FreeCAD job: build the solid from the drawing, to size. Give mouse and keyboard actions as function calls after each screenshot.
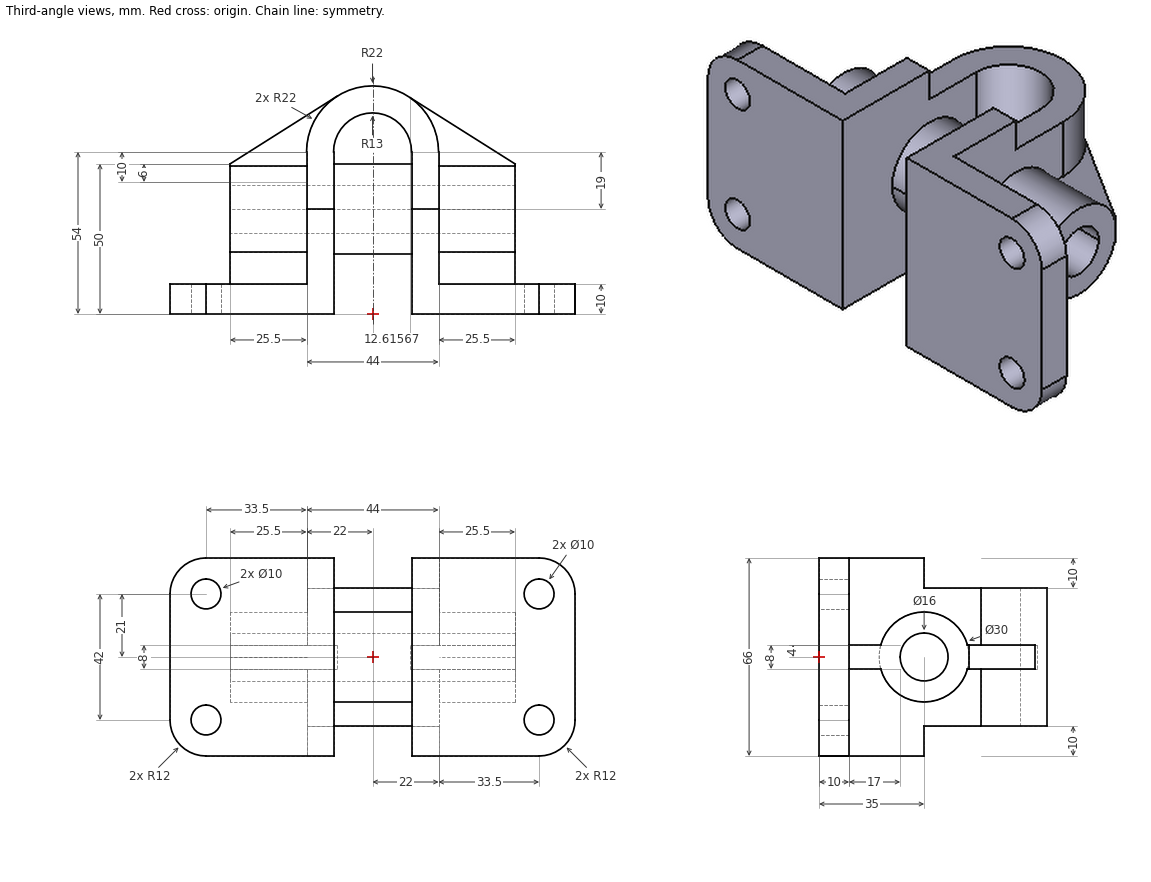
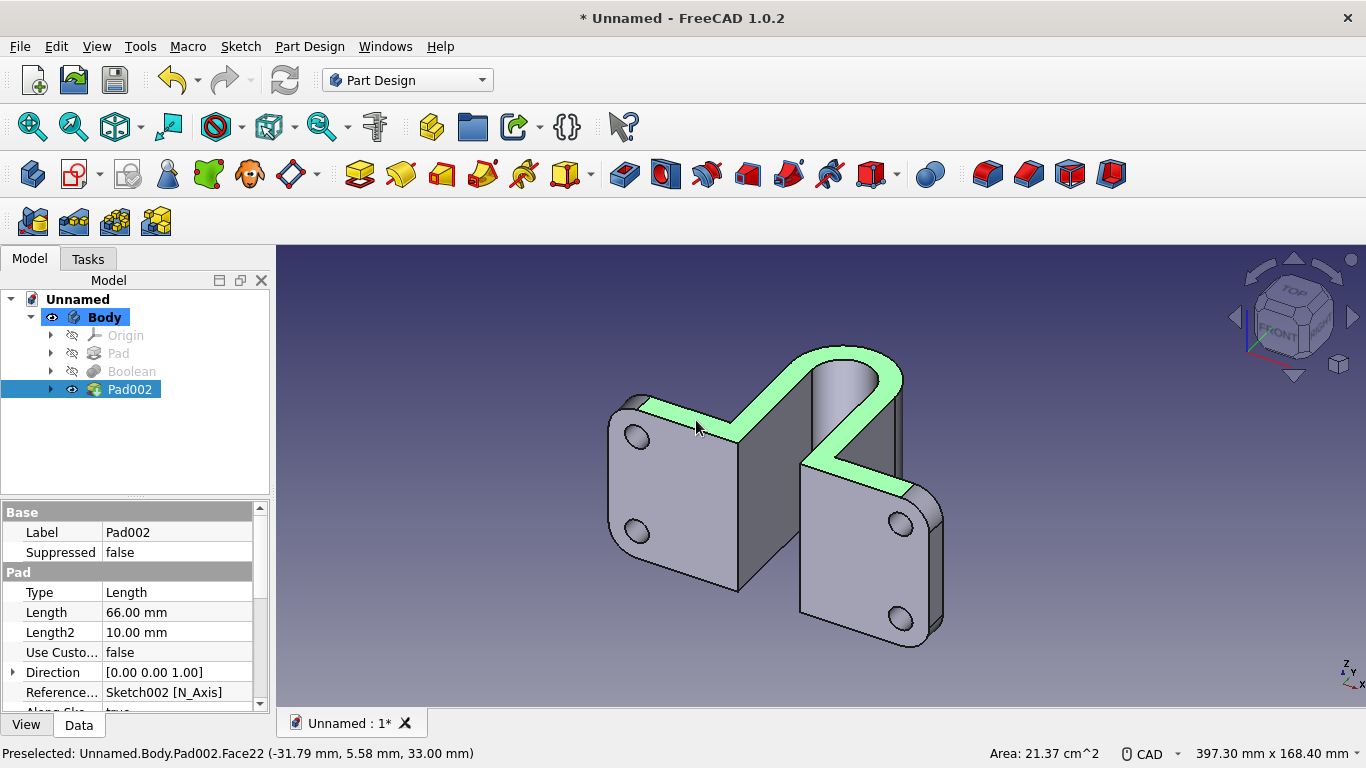
click(74, 174)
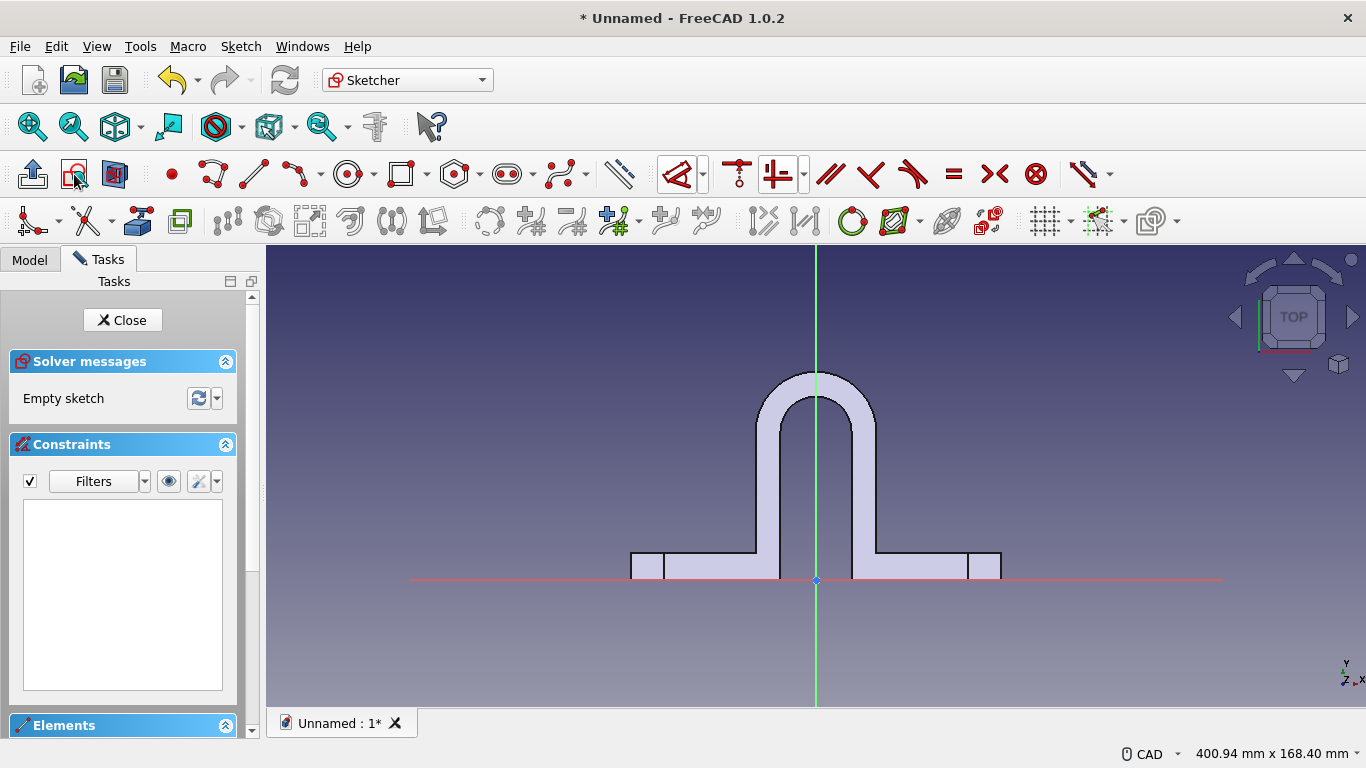
scroll(955, 476, up, 2)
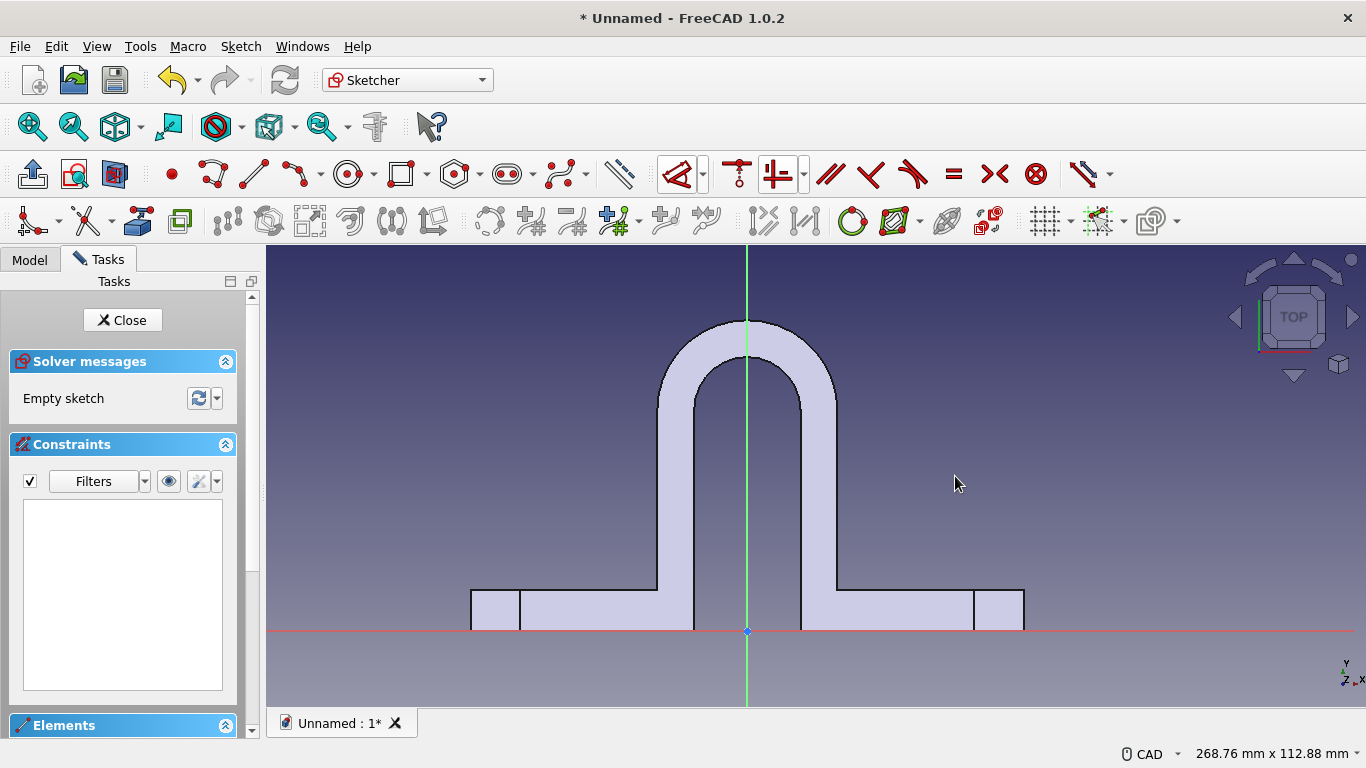
click(213, 174)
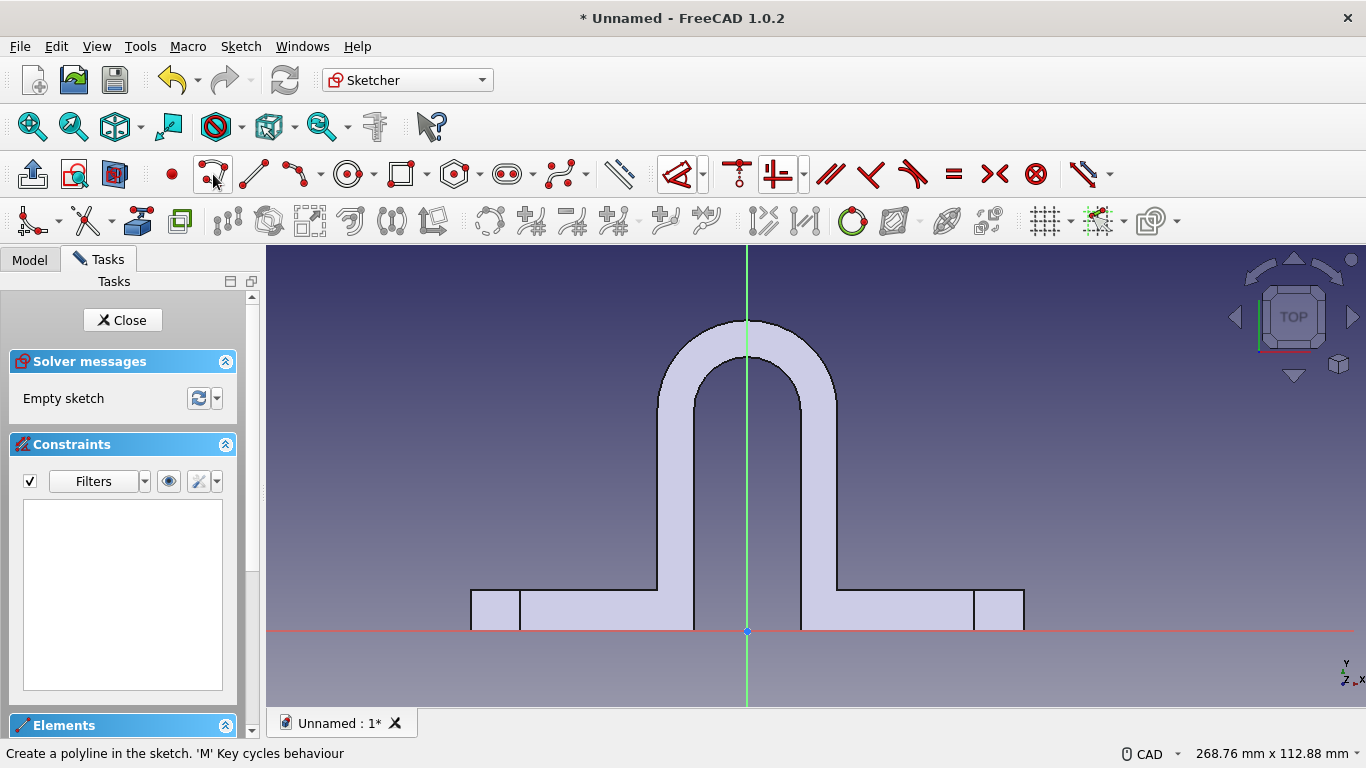
click(801, 410)
click(801, 488)
click(837, 488)
click(837, 410)
right_click(837, 410)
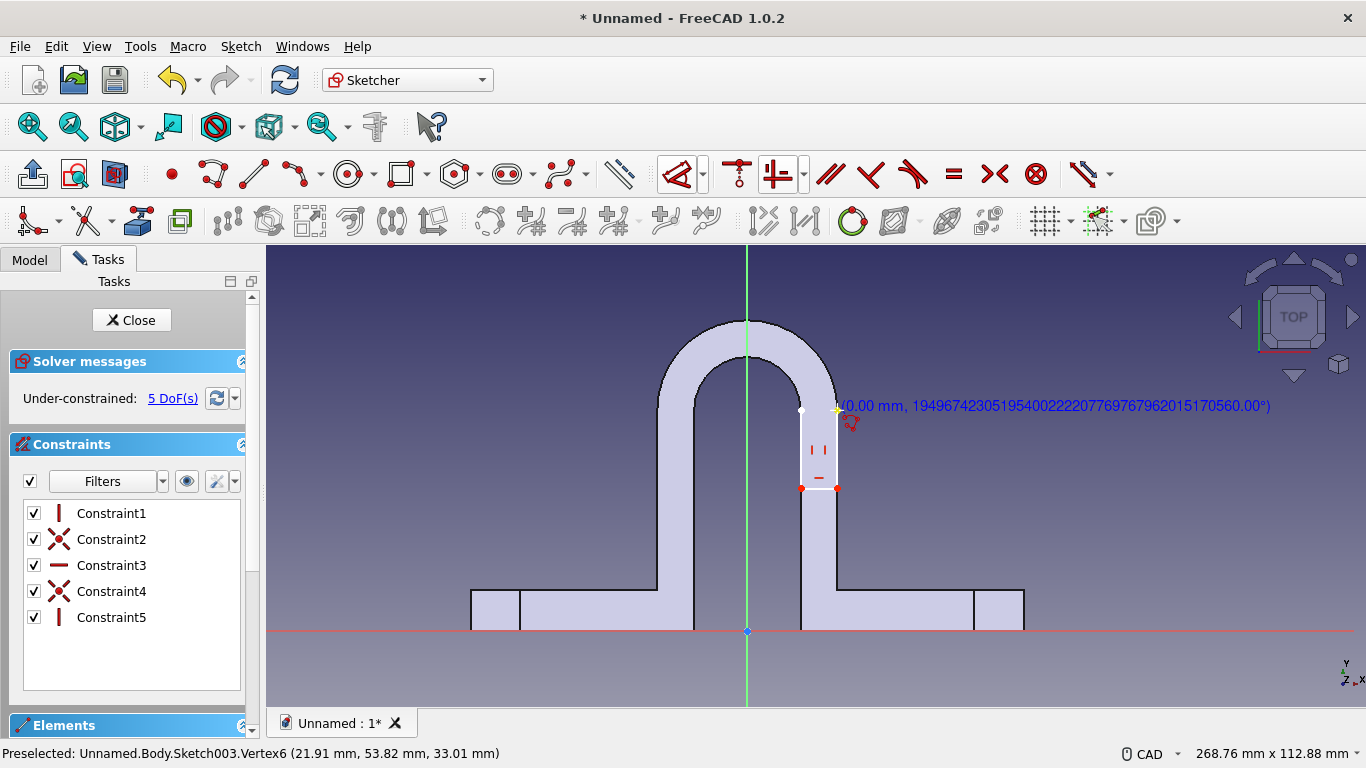
click(657, 410)
click(657, 488)
click(694, 488)
click(694, 410)
right_click(694, 410)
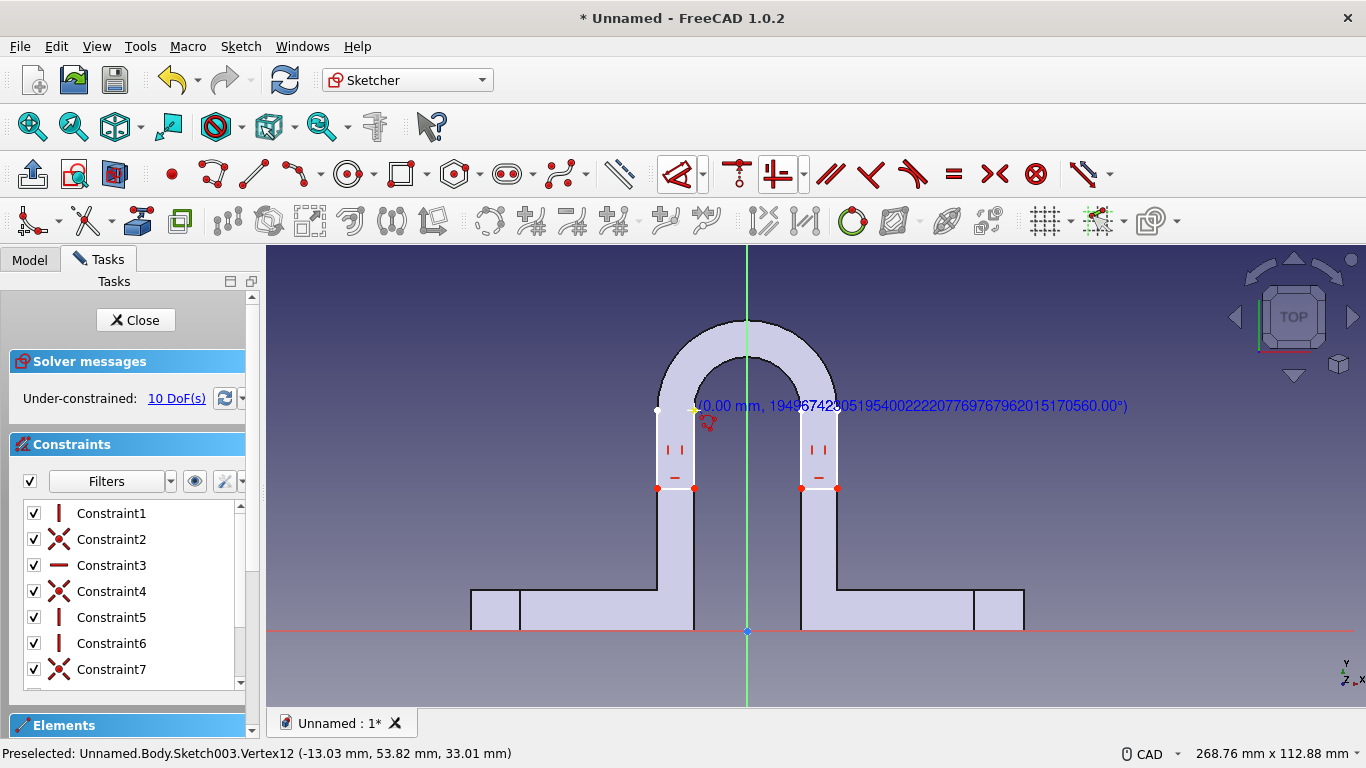
click(294, 174)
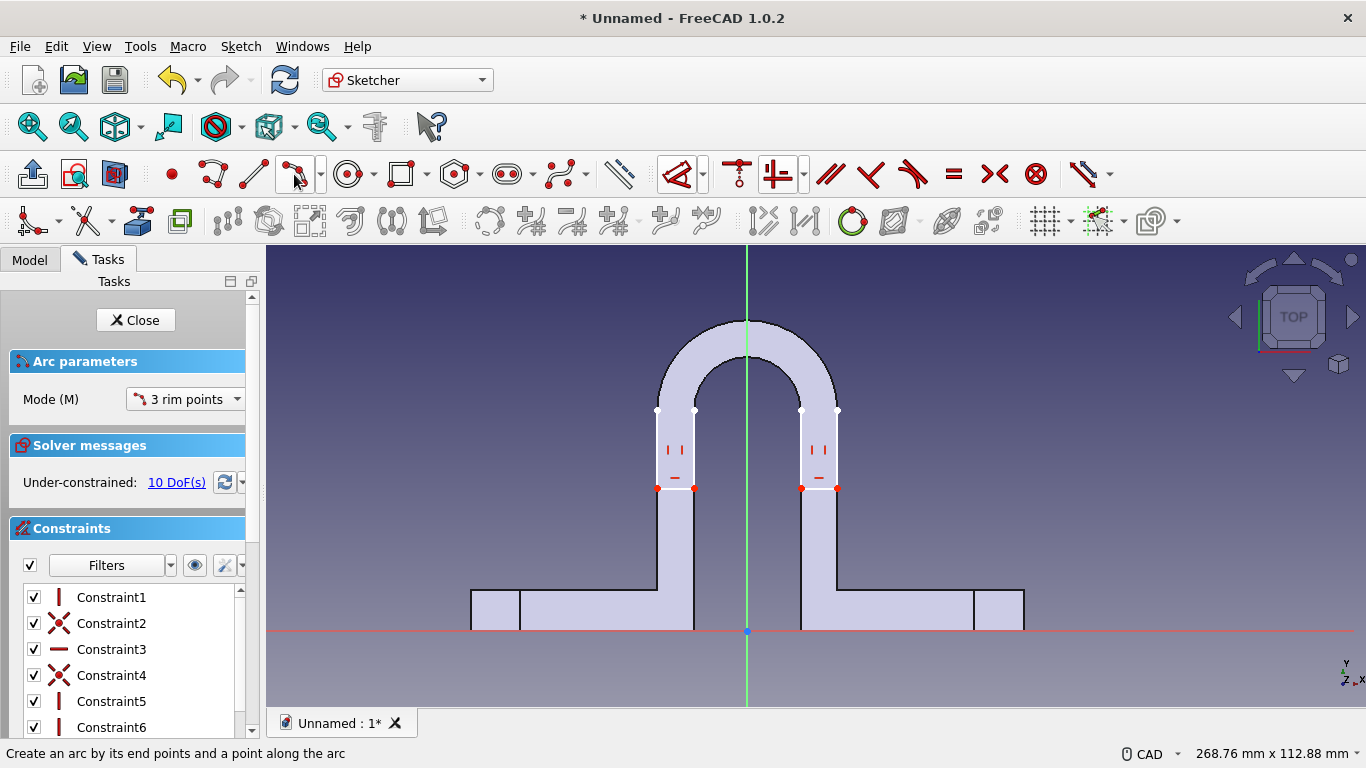
click(837, 411)
click(657, 411)
click(775, 325)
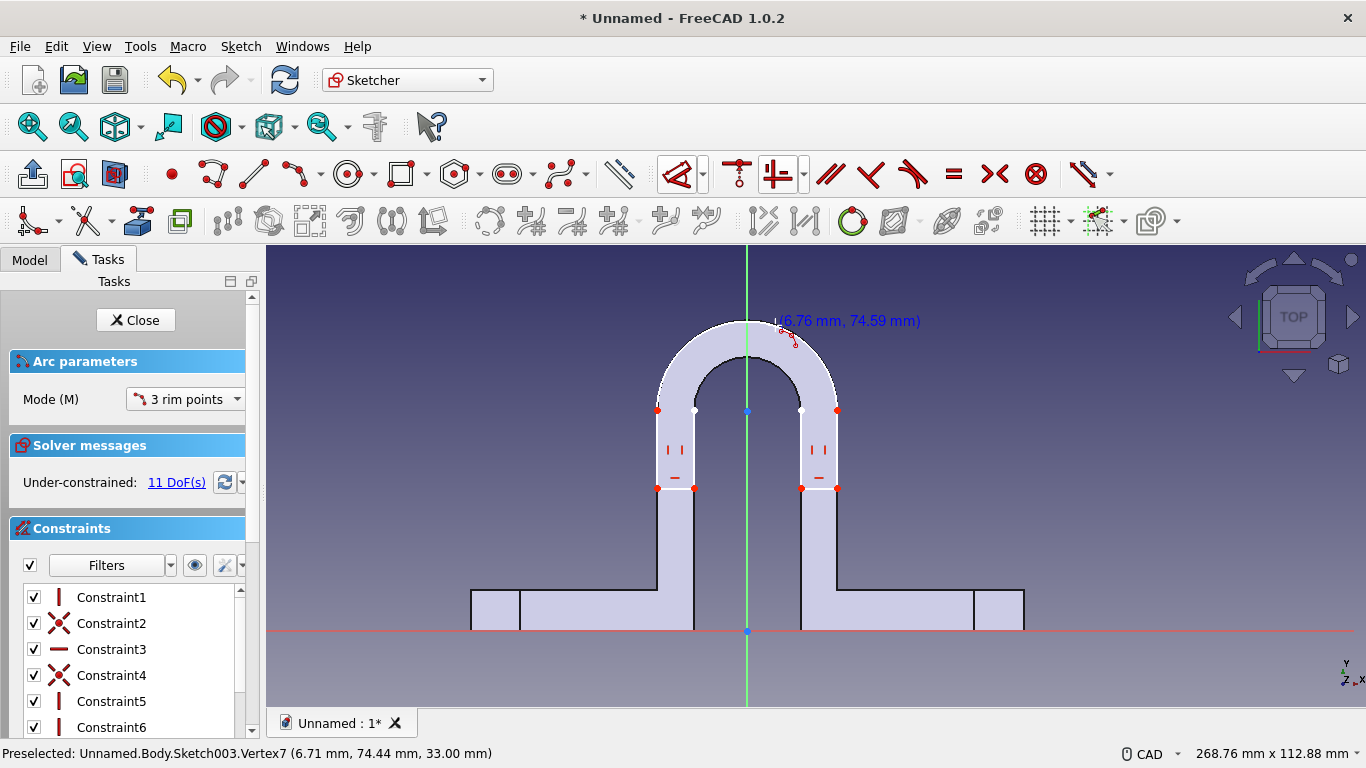
click(694, 411)
click(801, 411)
click(764, 360)
key(Escape)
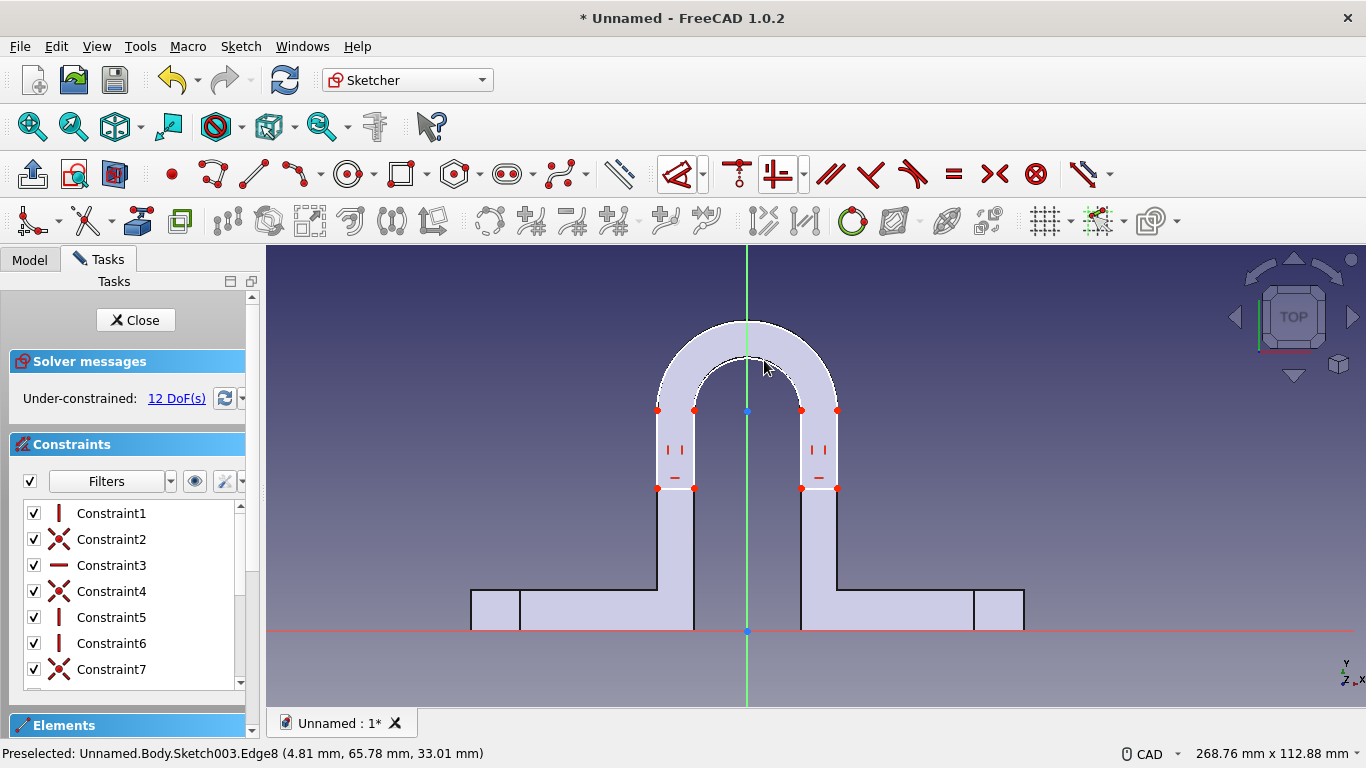
click(801, 434)